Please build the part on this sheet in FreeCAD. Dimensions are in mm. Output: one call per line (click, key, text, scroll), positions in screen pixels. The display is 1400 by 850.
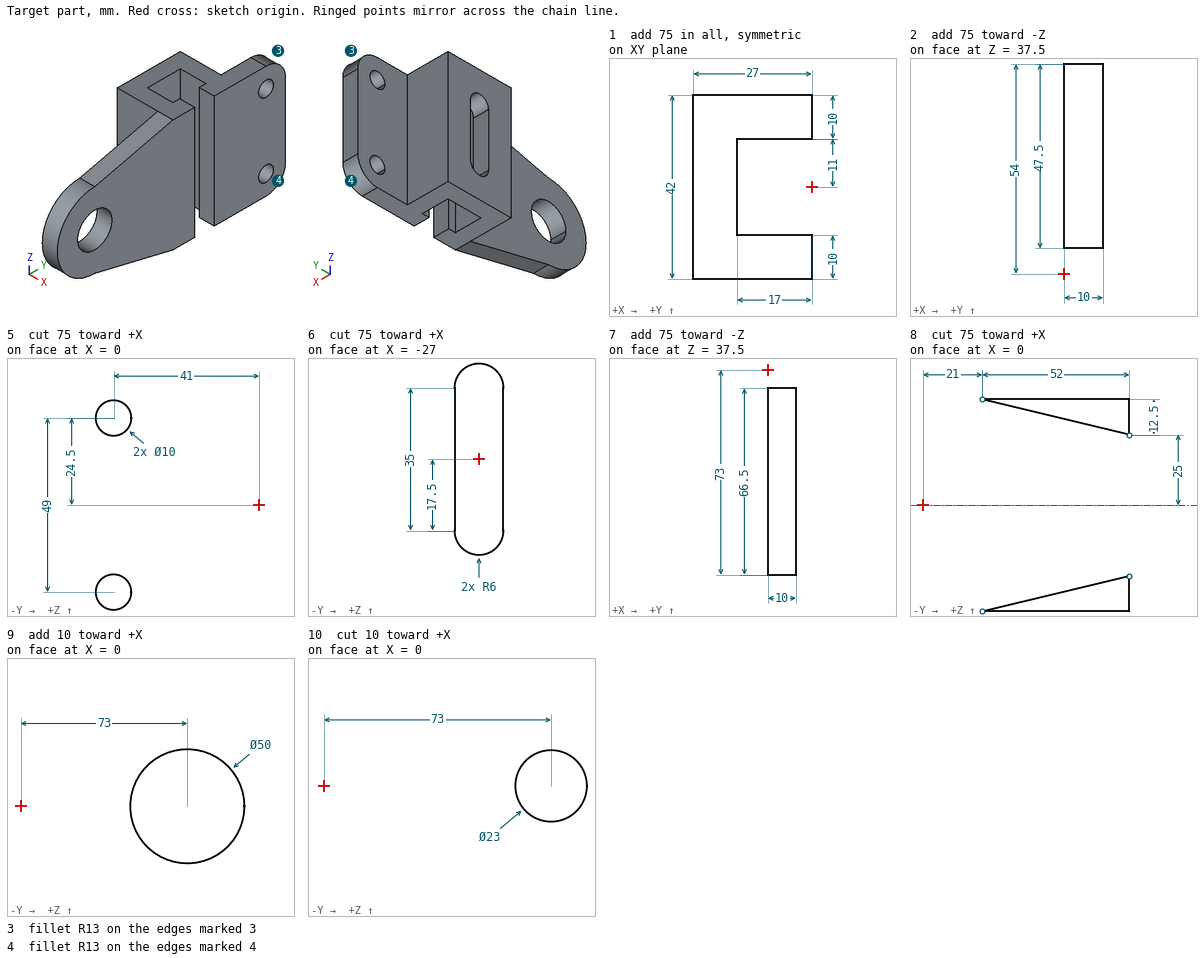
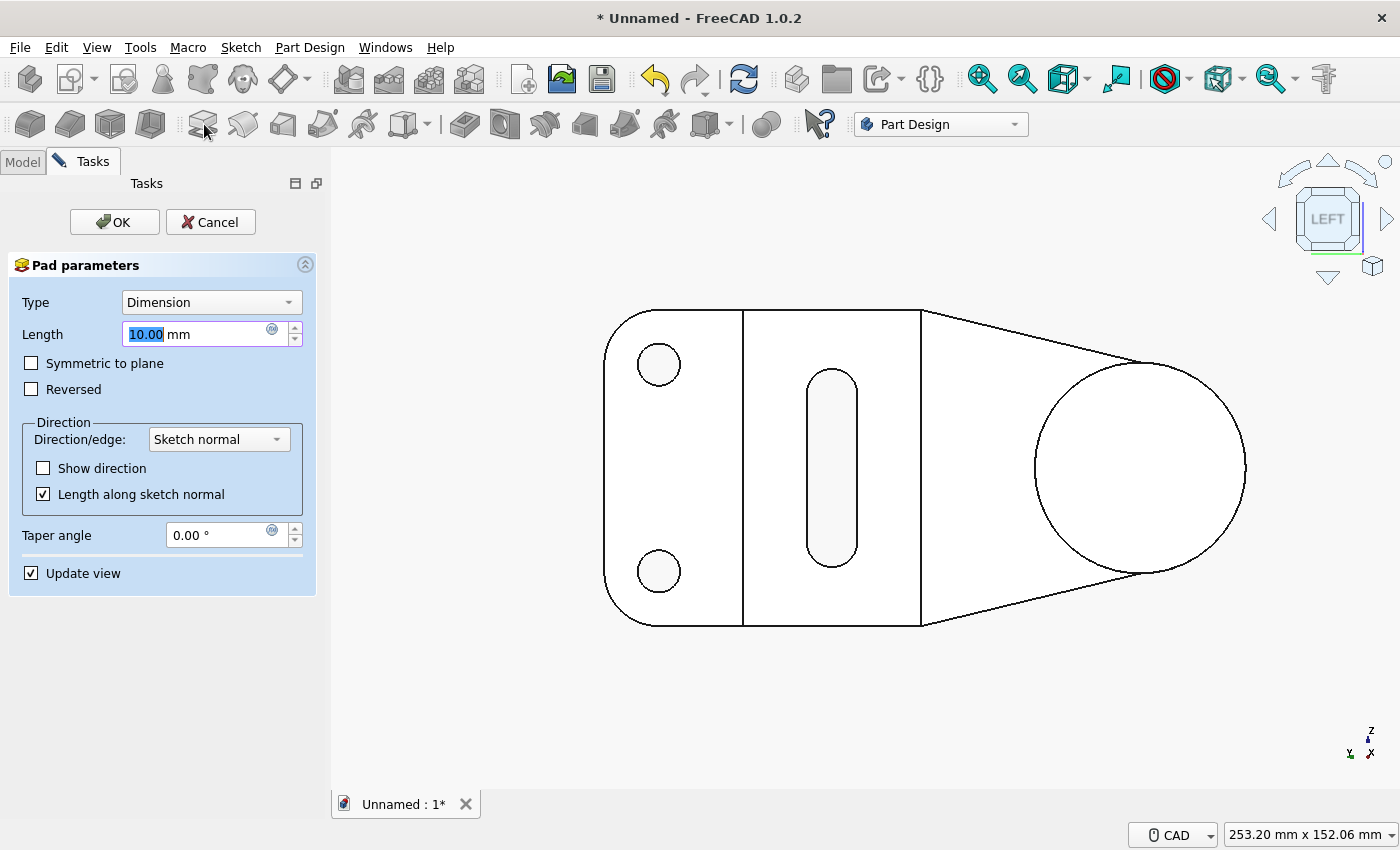
text(10)
key(Tab)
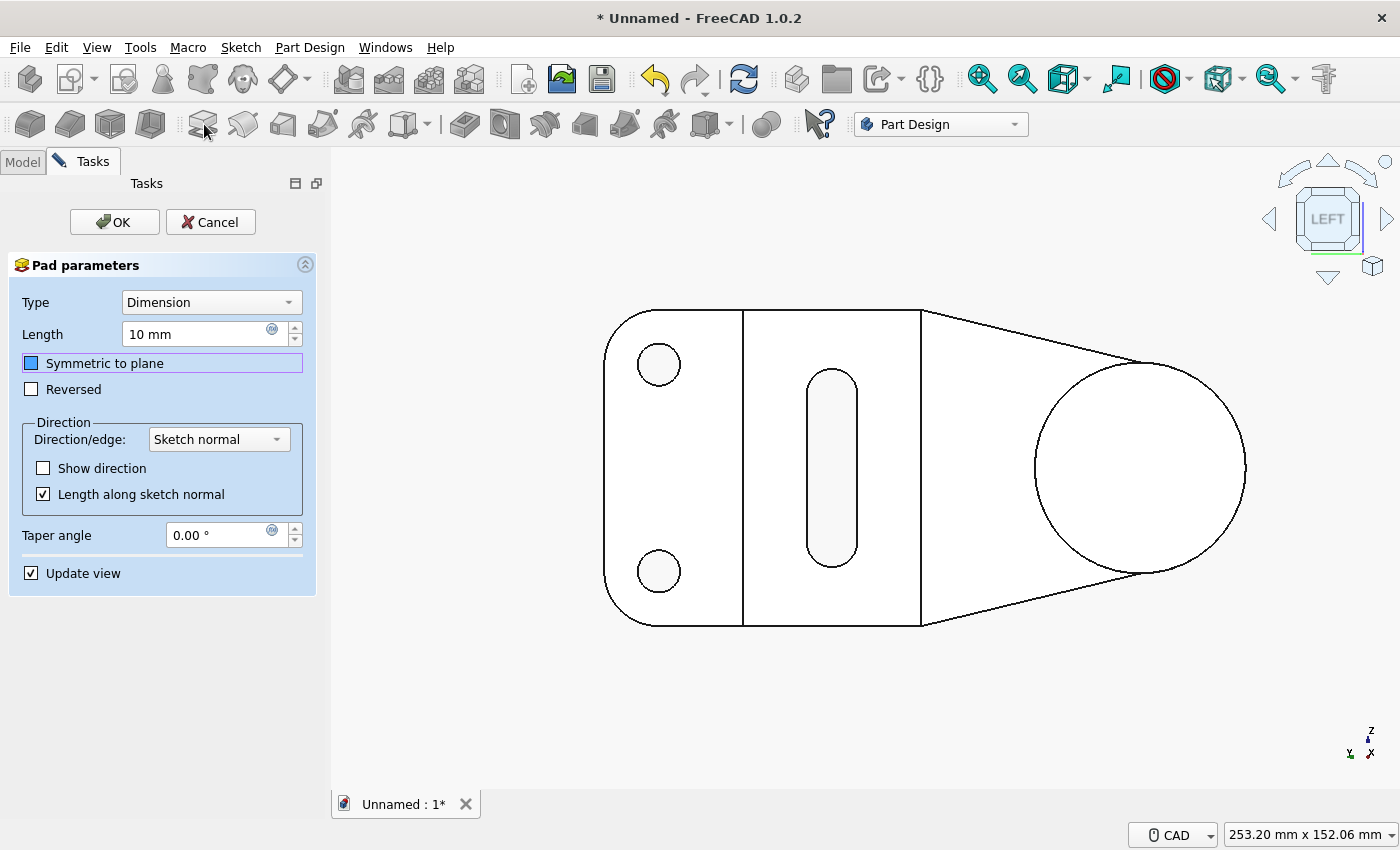
click(30, 389)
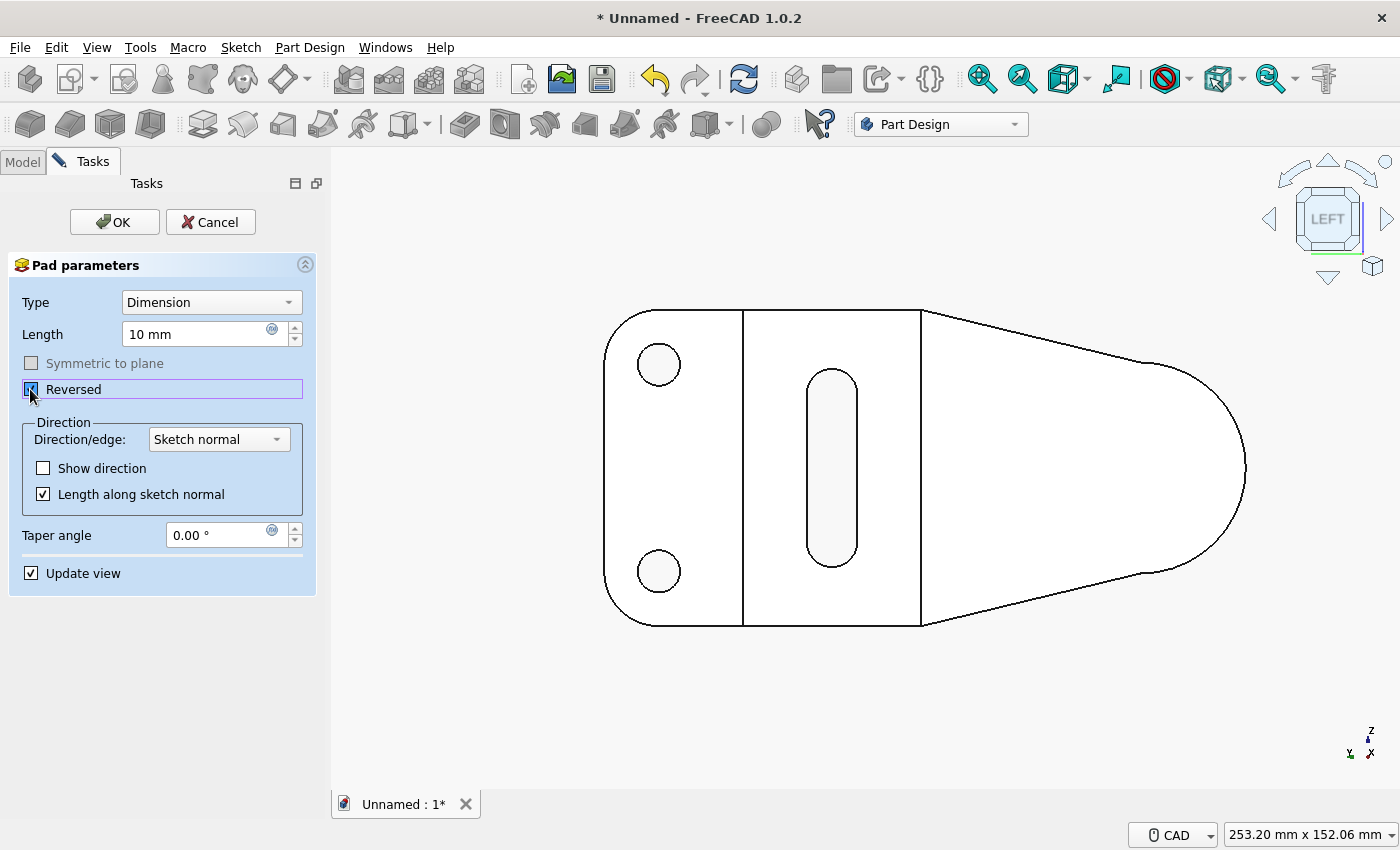
click(115, 222)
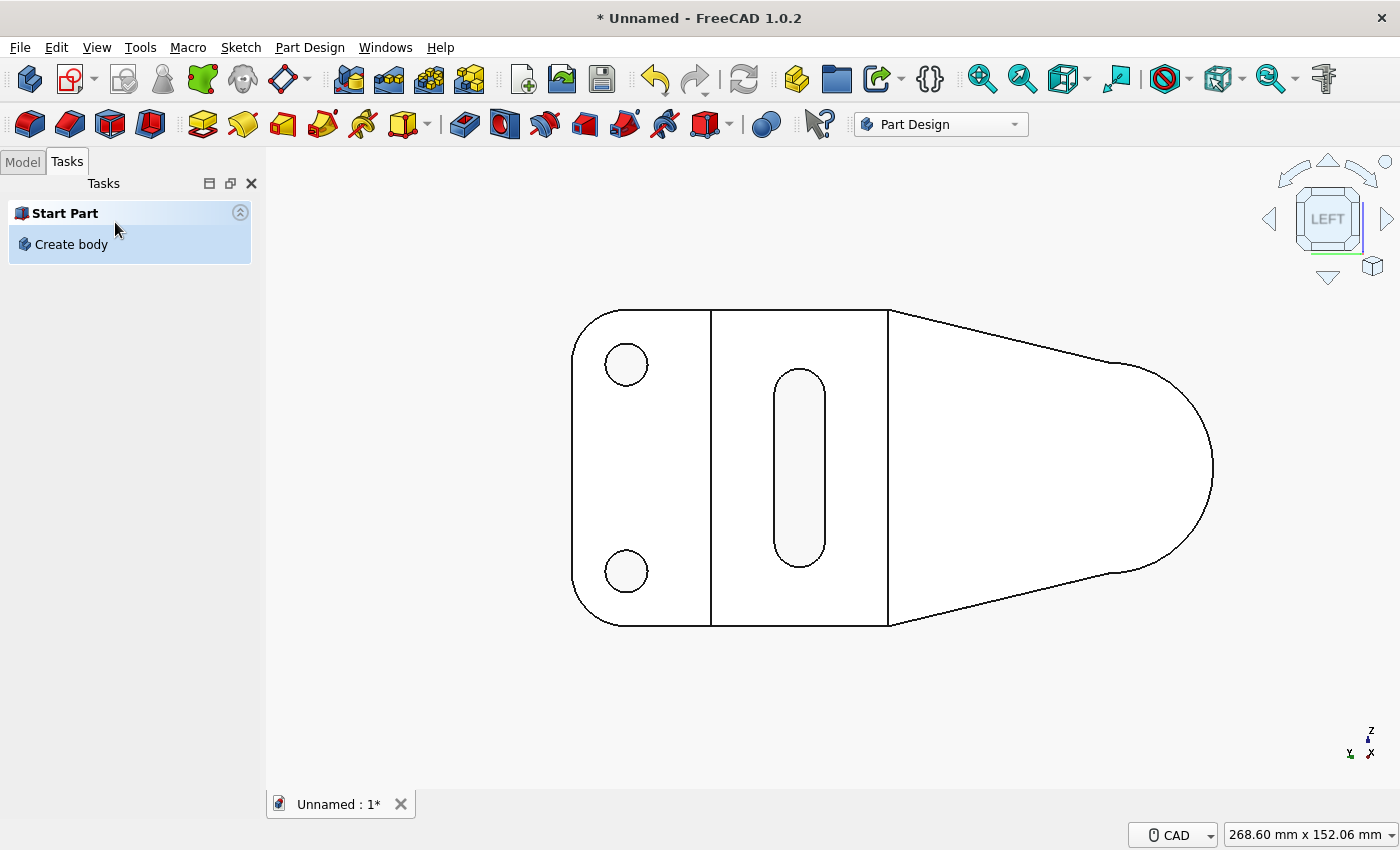
click(1004, 467)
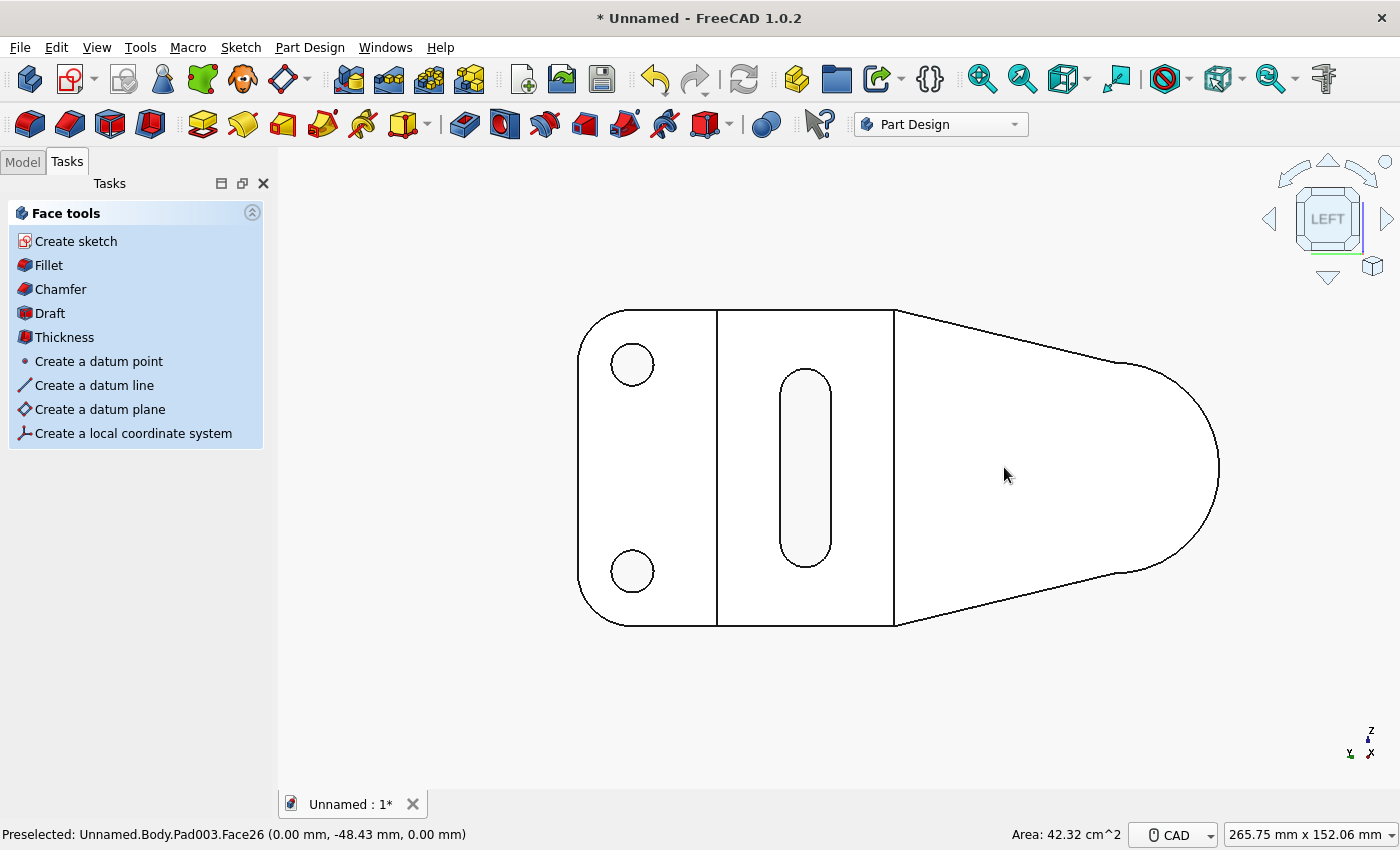
click(70, 80)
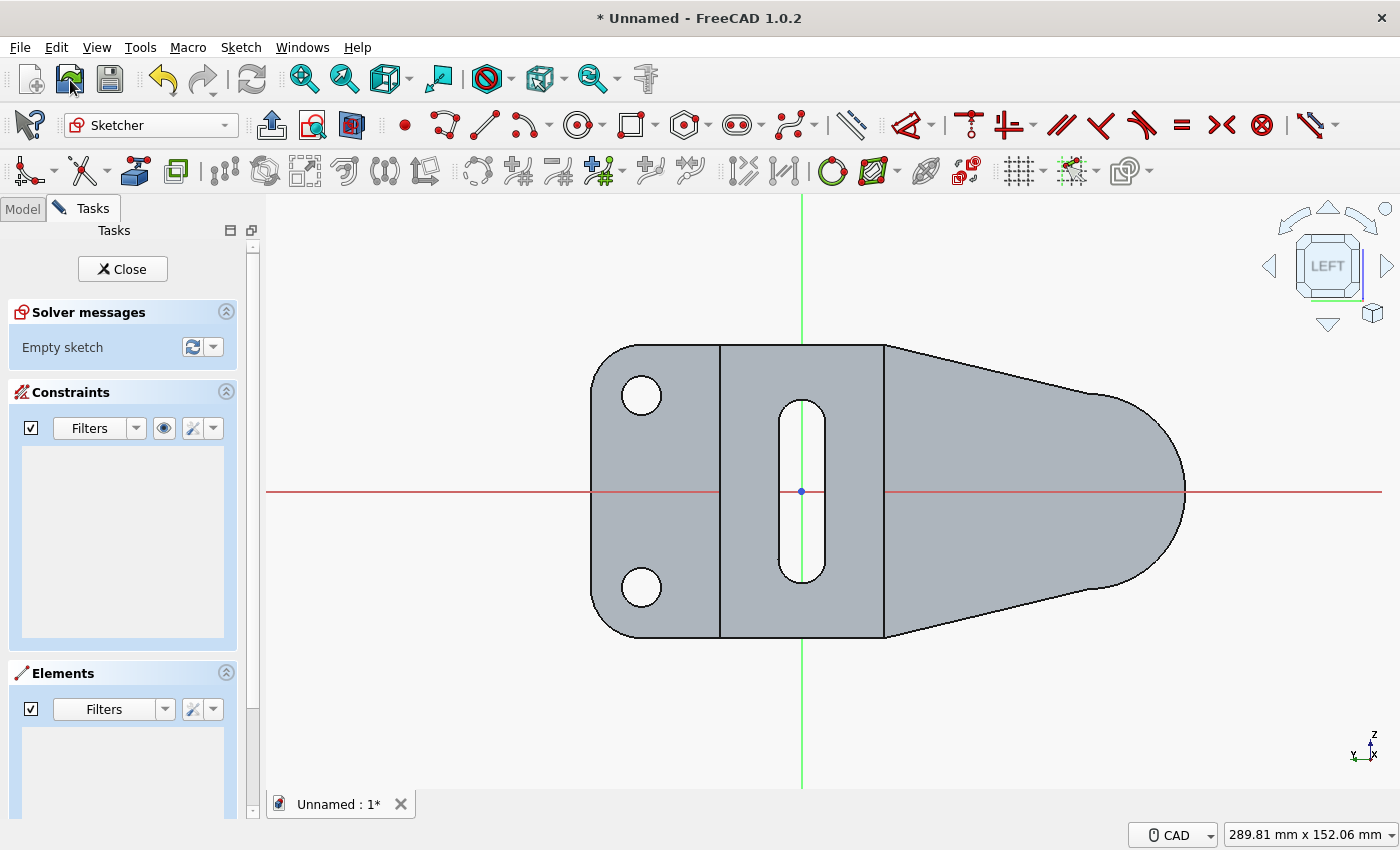
scroll(1193, 492, up, 7)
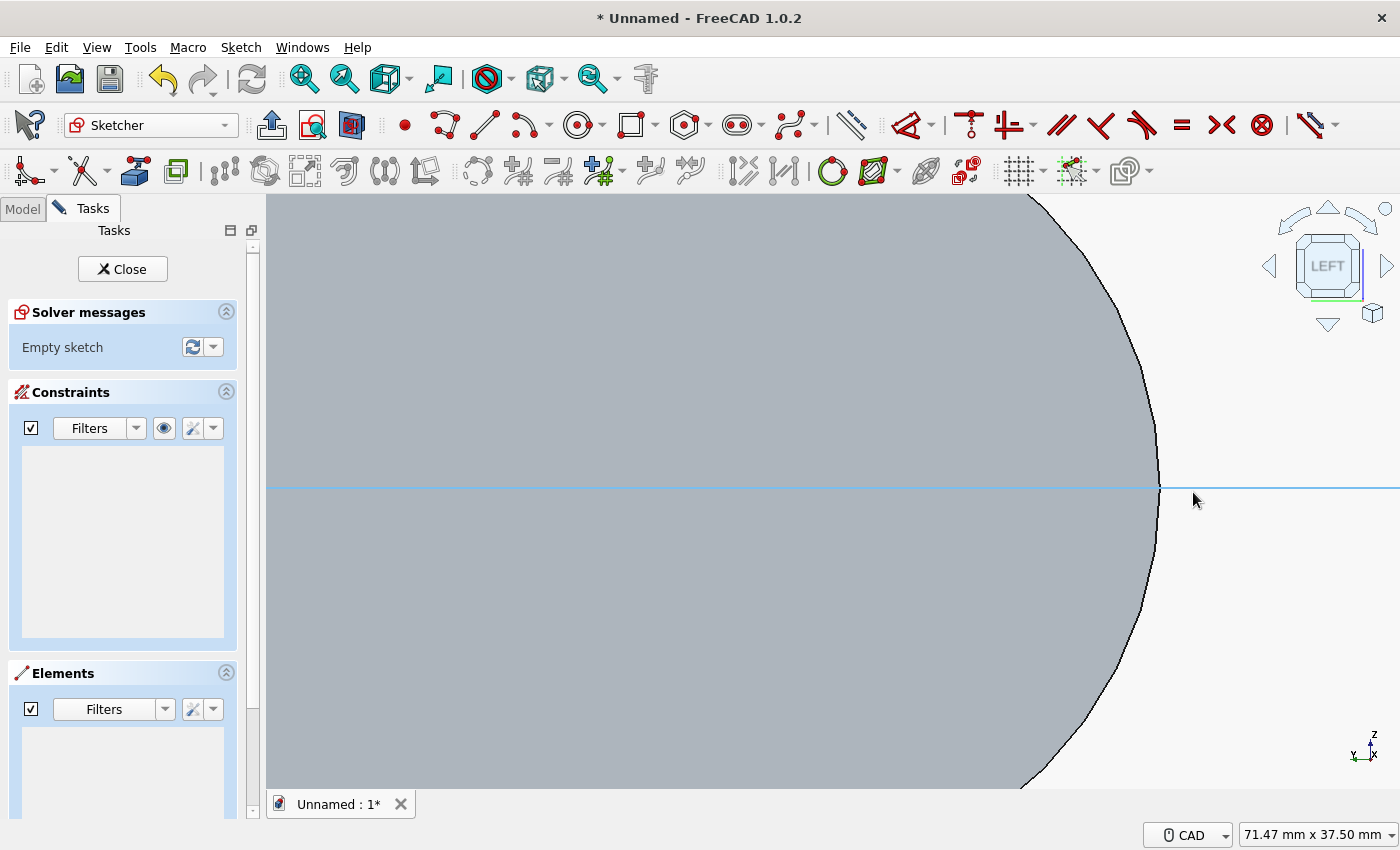
click(578, 126)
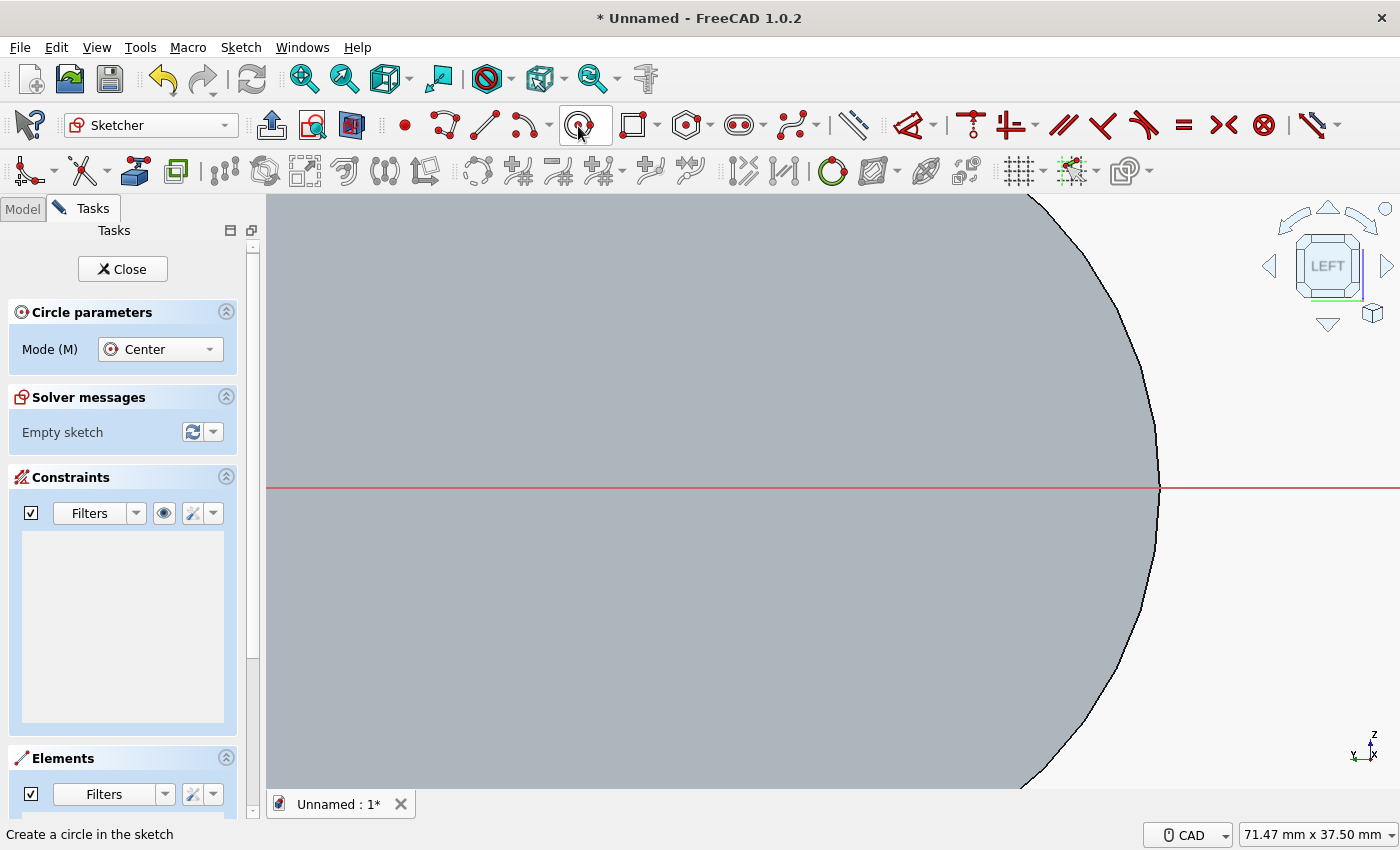
click(763, 488)
click(892, 359)
key(Escape)